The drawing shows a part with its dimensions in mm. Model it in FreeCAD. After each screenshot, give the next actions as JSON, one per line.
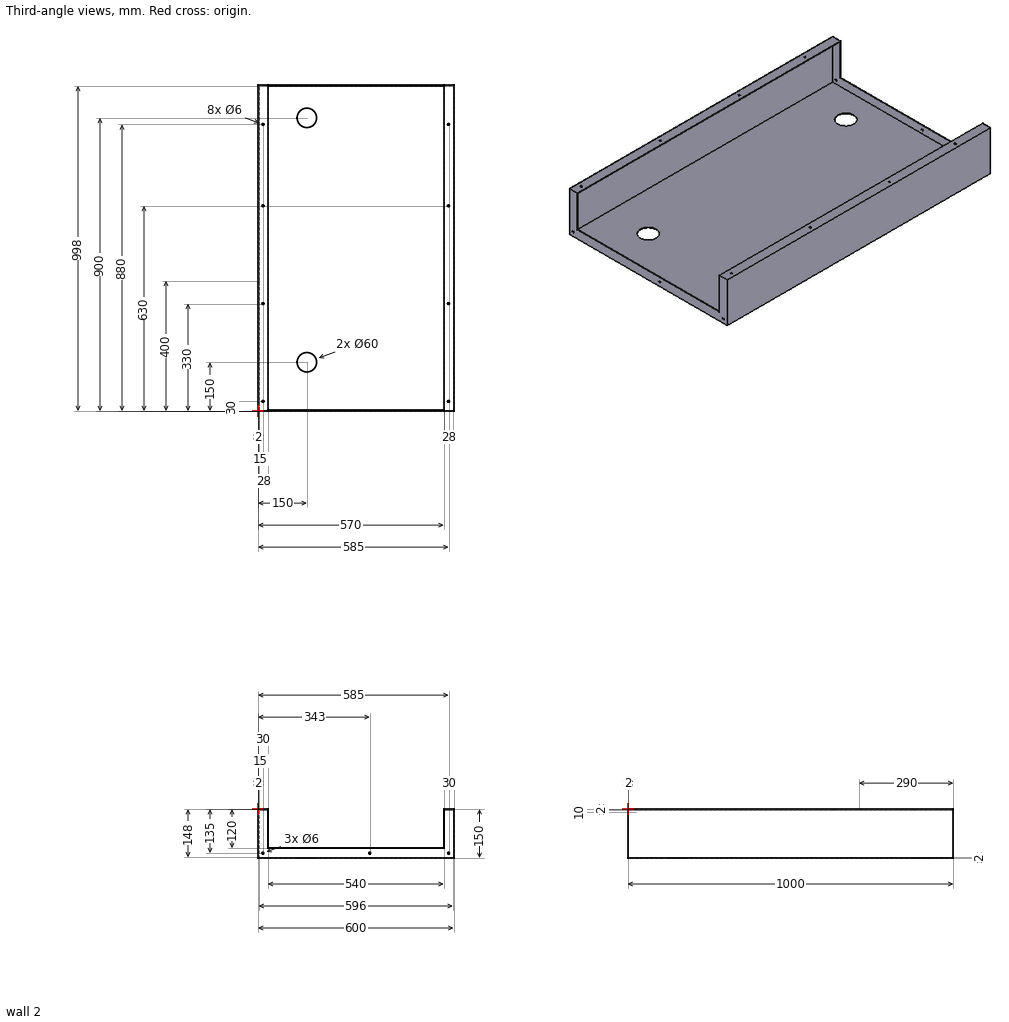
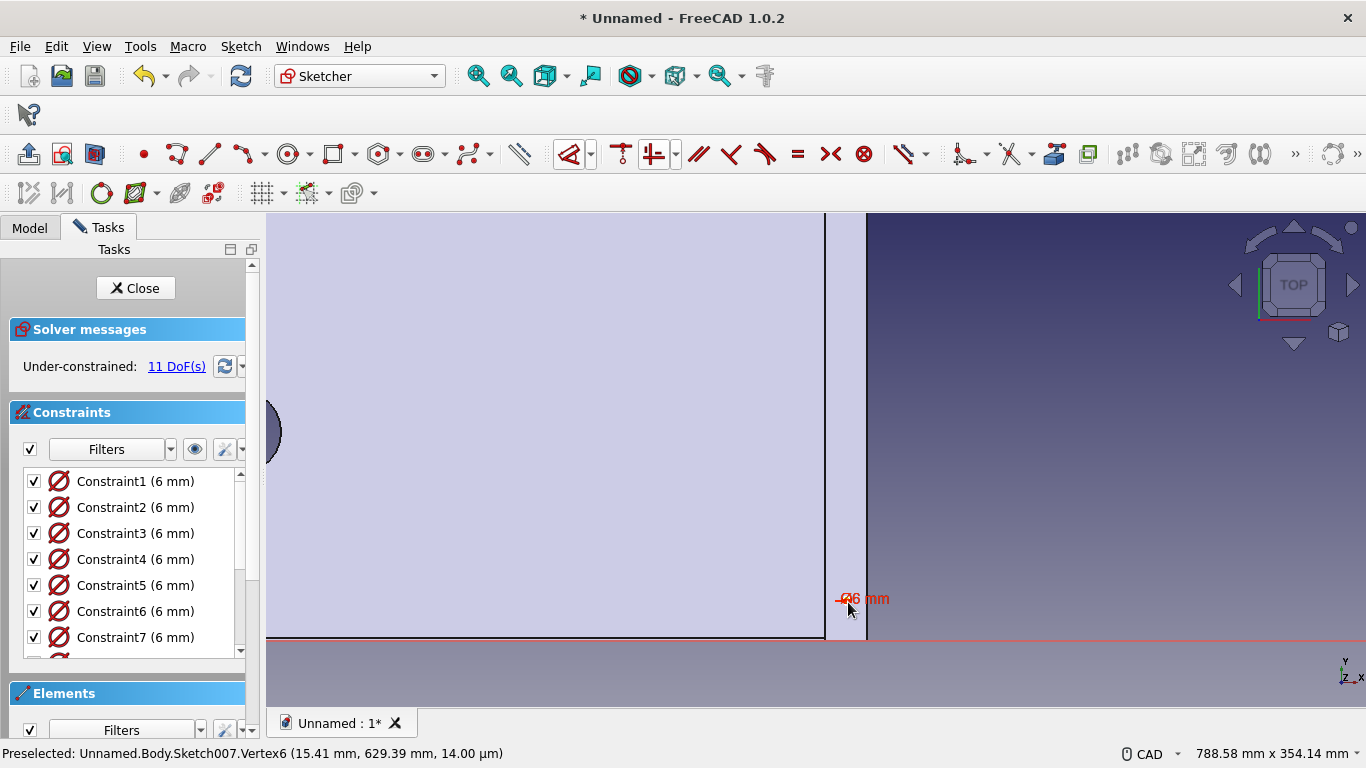
{"action": "left_click", "coordinate": [847, 601]}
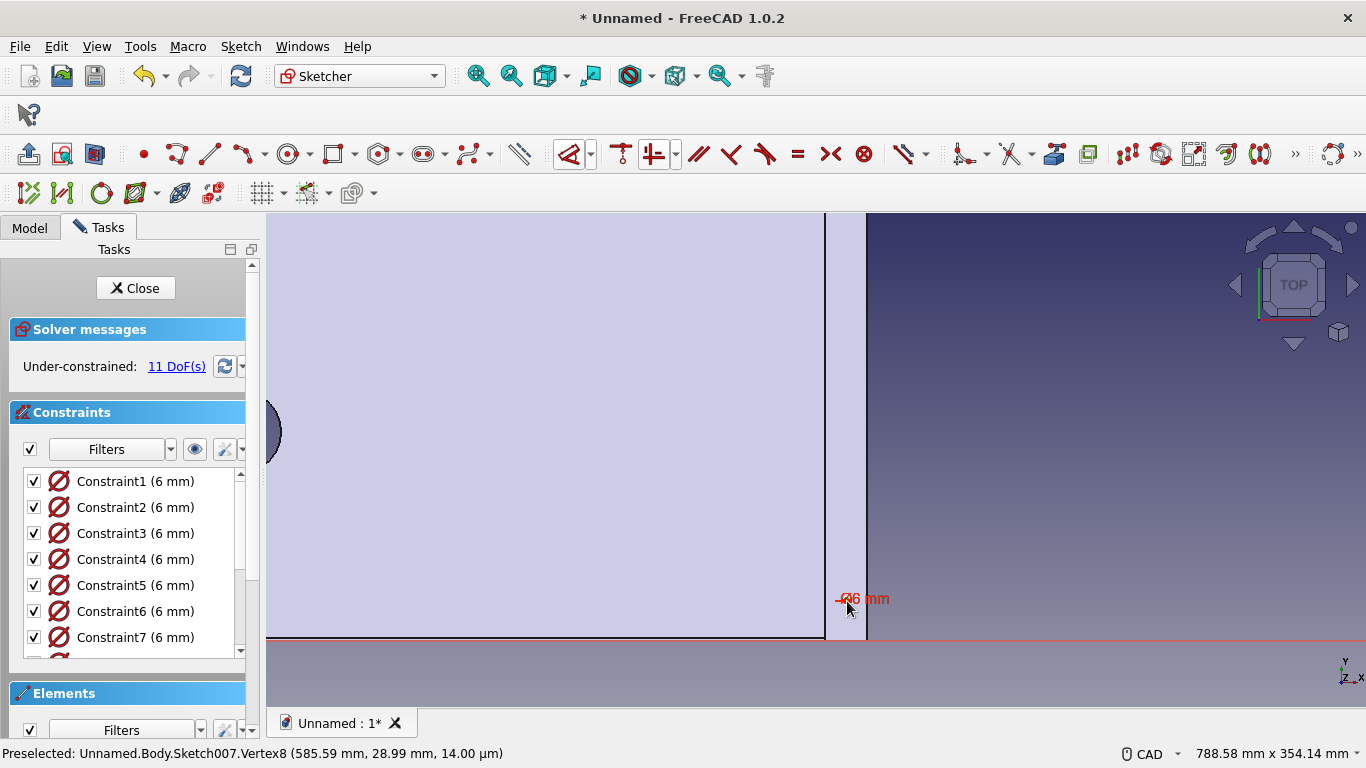
{"action": "left_click", "coordinate": [590, 154]}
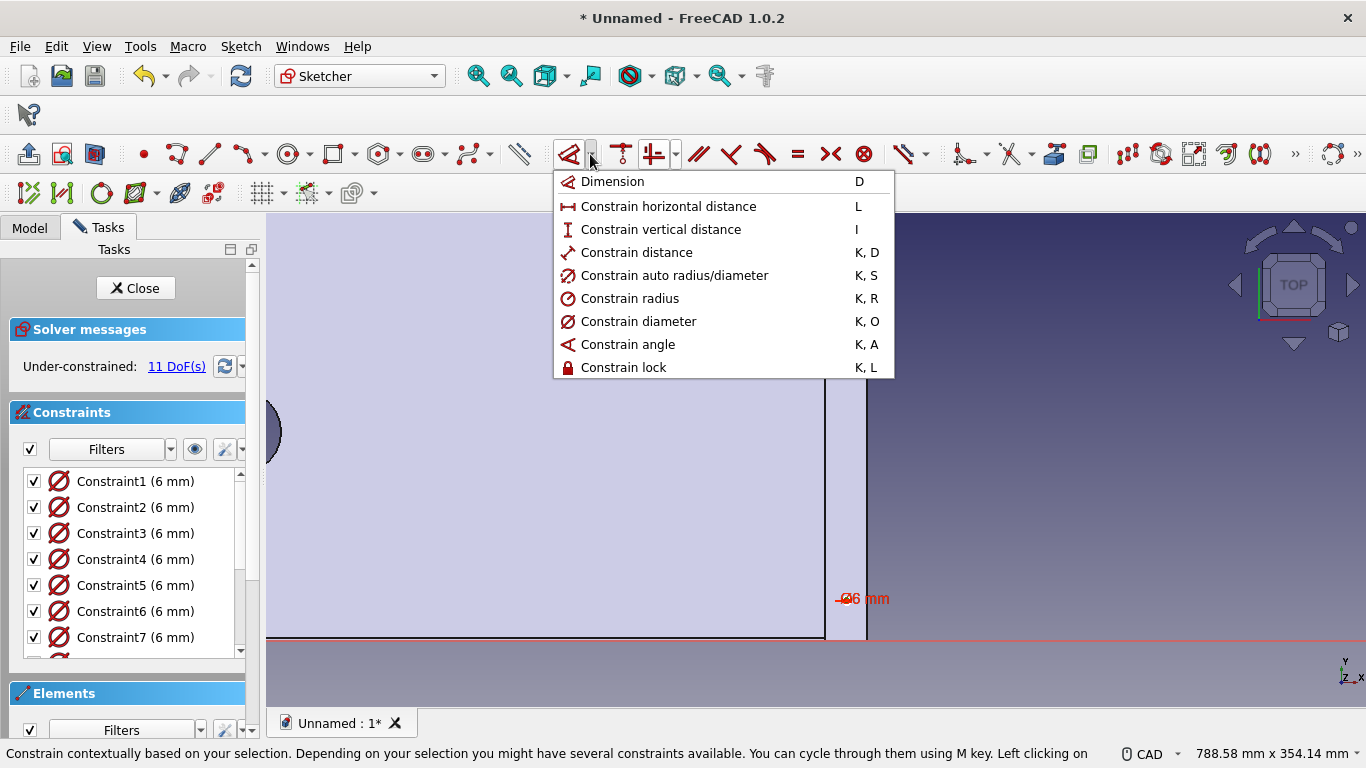
{"action": "left_click", "coordinate": [724, 230]}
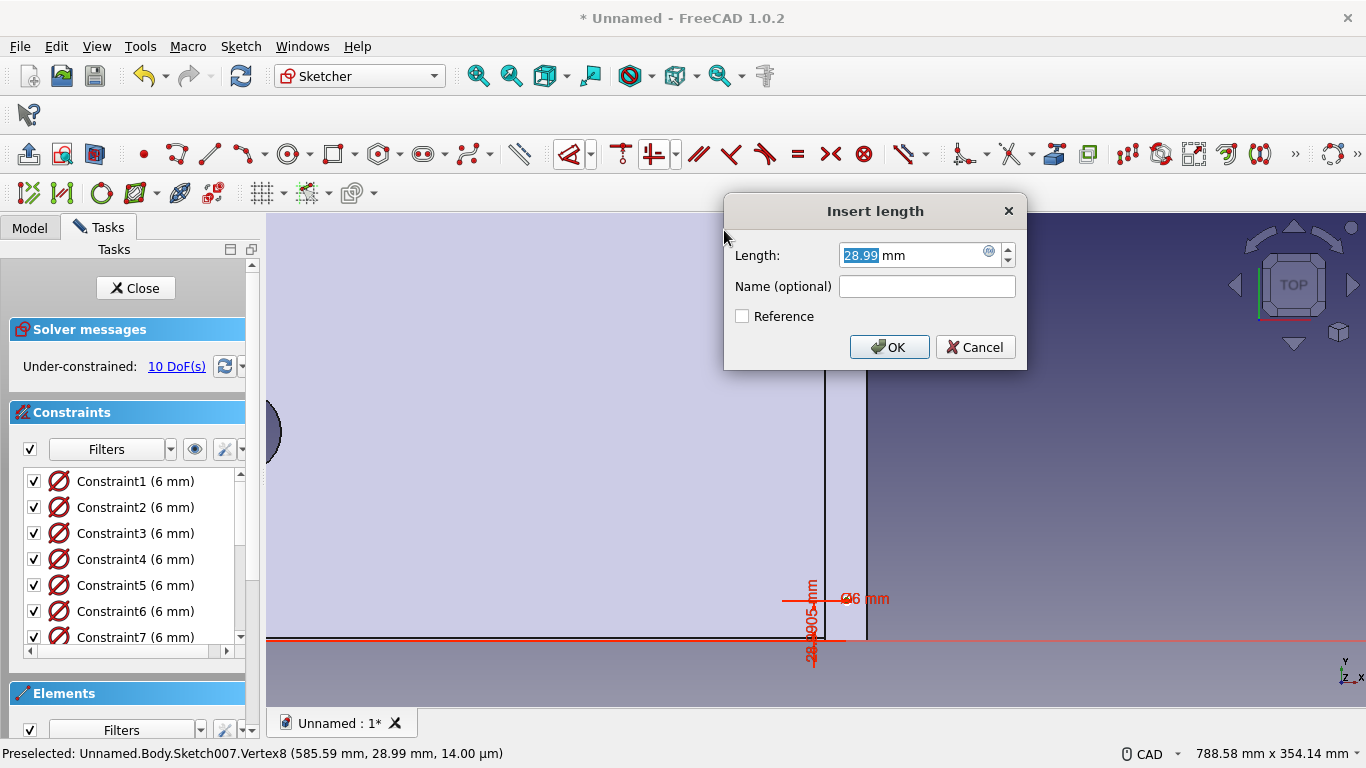
{"action": "type", "text": "30"}
{"action": "key", "text": "Return"}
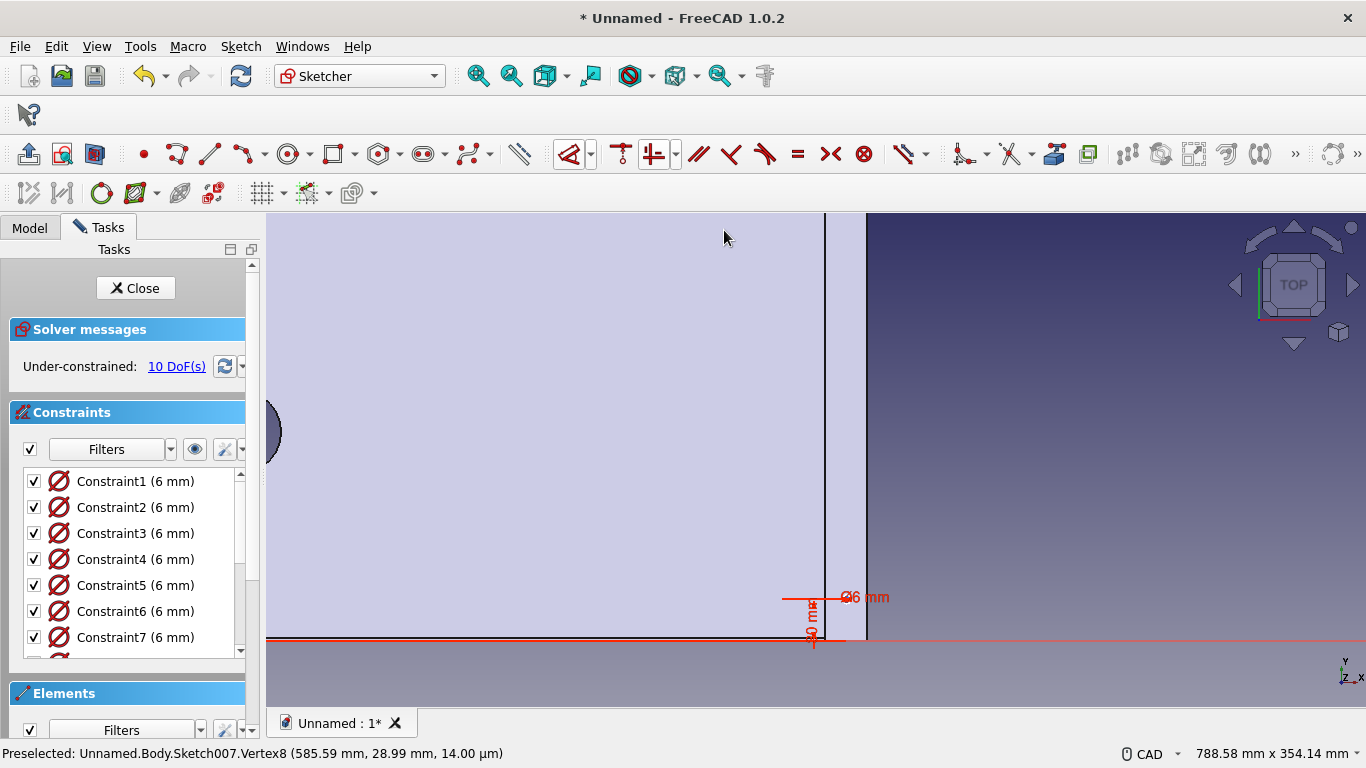
{"action": "scroll", "coordinate": [848, 602], "scroll_direction": "down", "scroll_amount": 7}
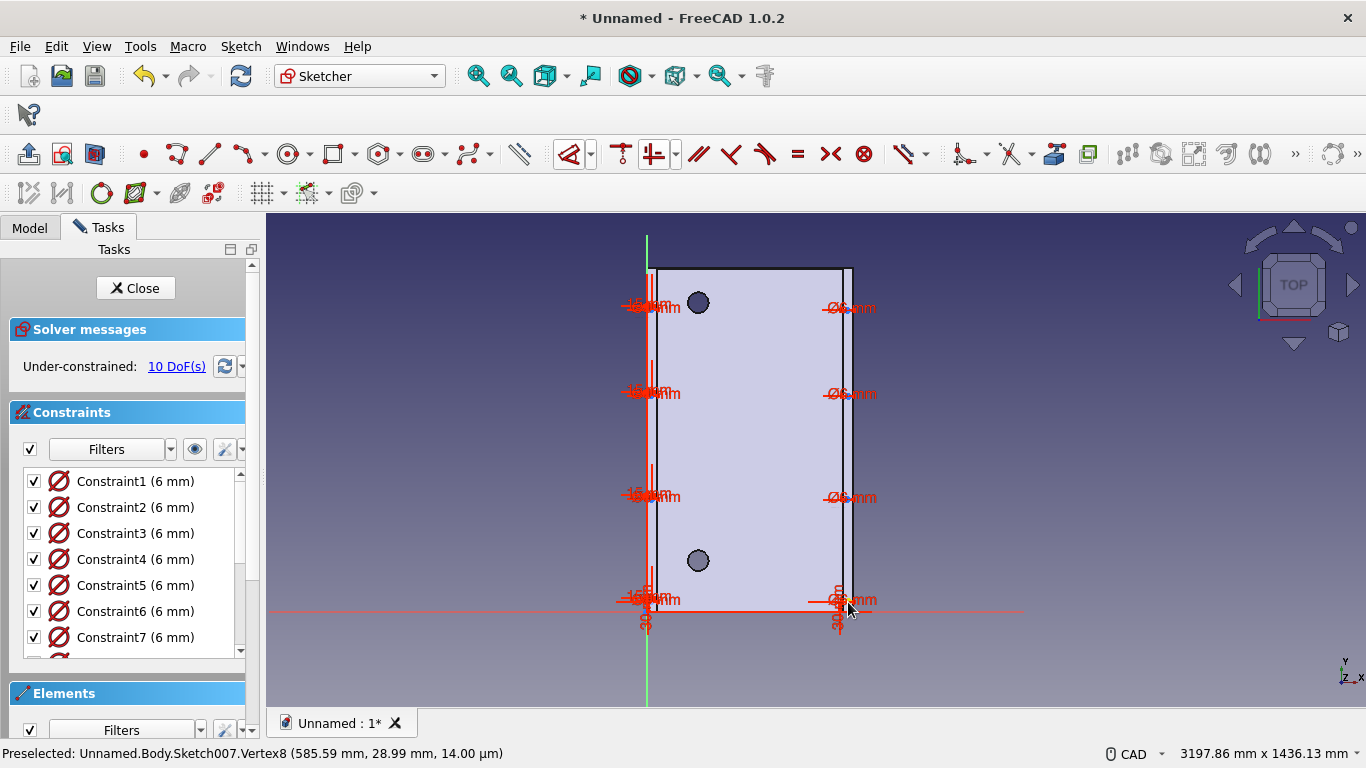
{"action": "left_click", "coordinate": [652, 310]}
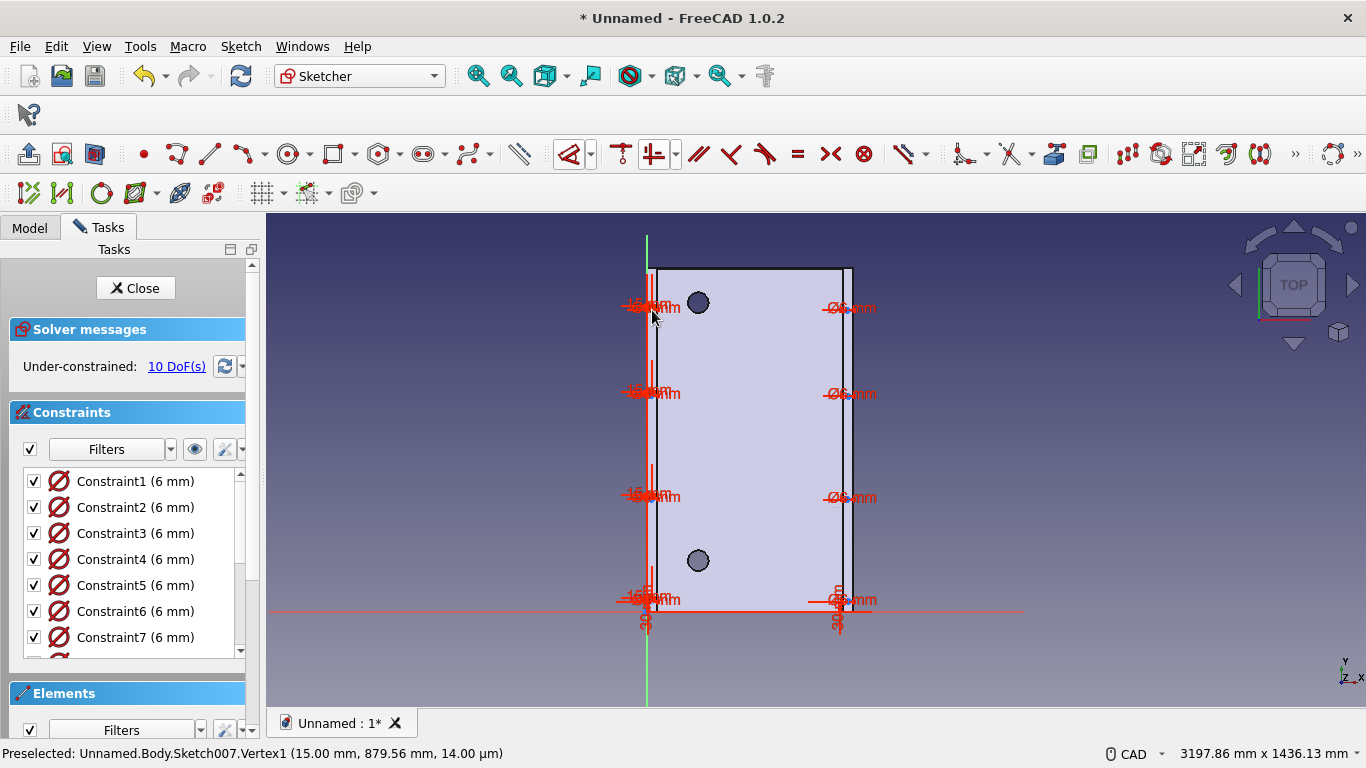
{"action": "left_click", "coordinate": [590, 154]}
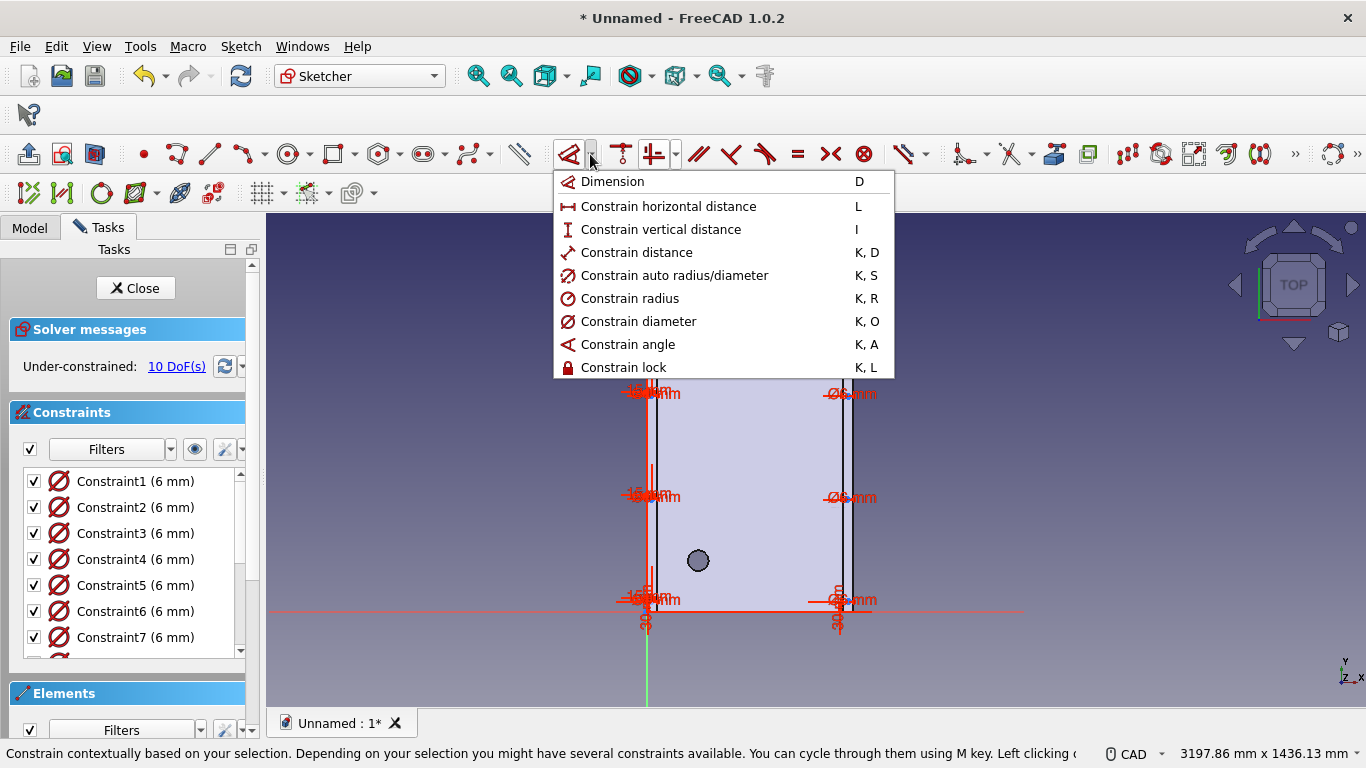
{"action": "left_click", "coordinate": [724, 230]}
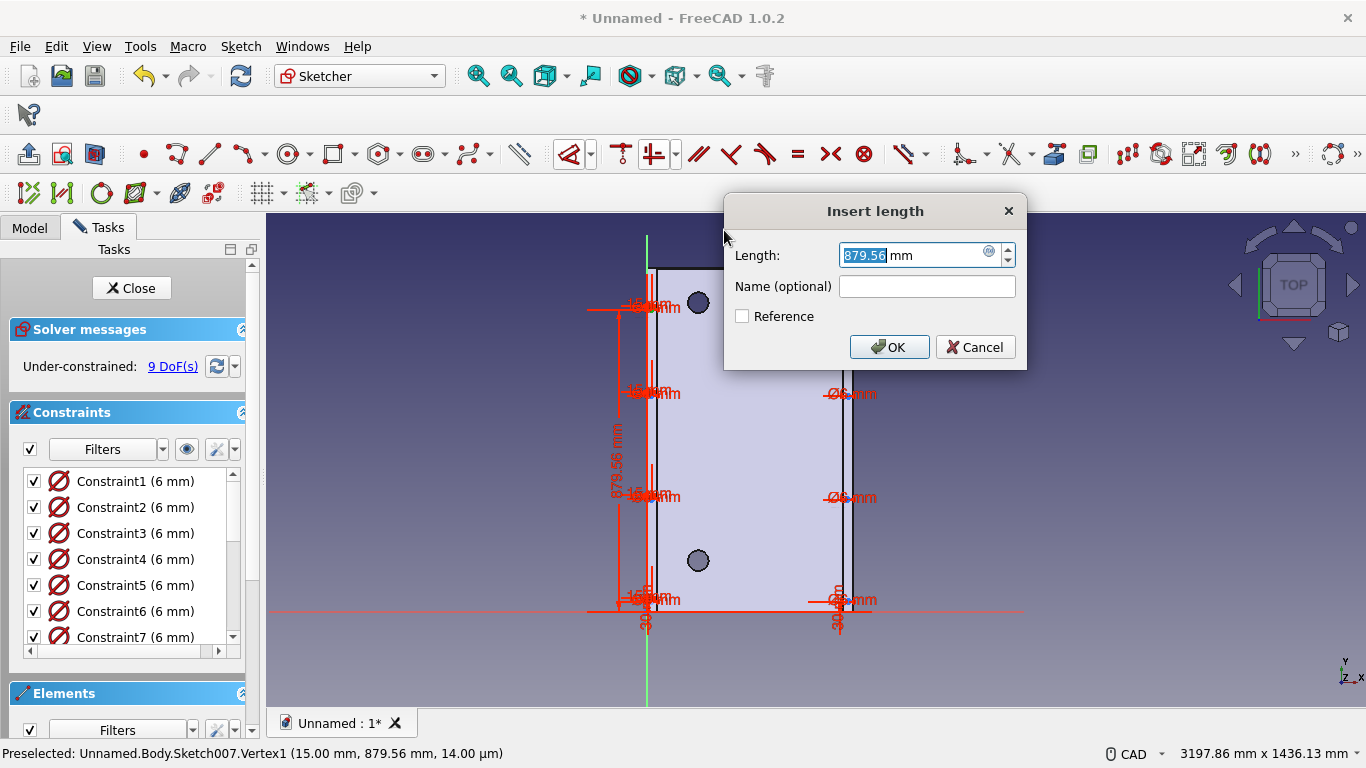
{"action": "type", "text": "880"}
{"action": "key", "text": "Return"}